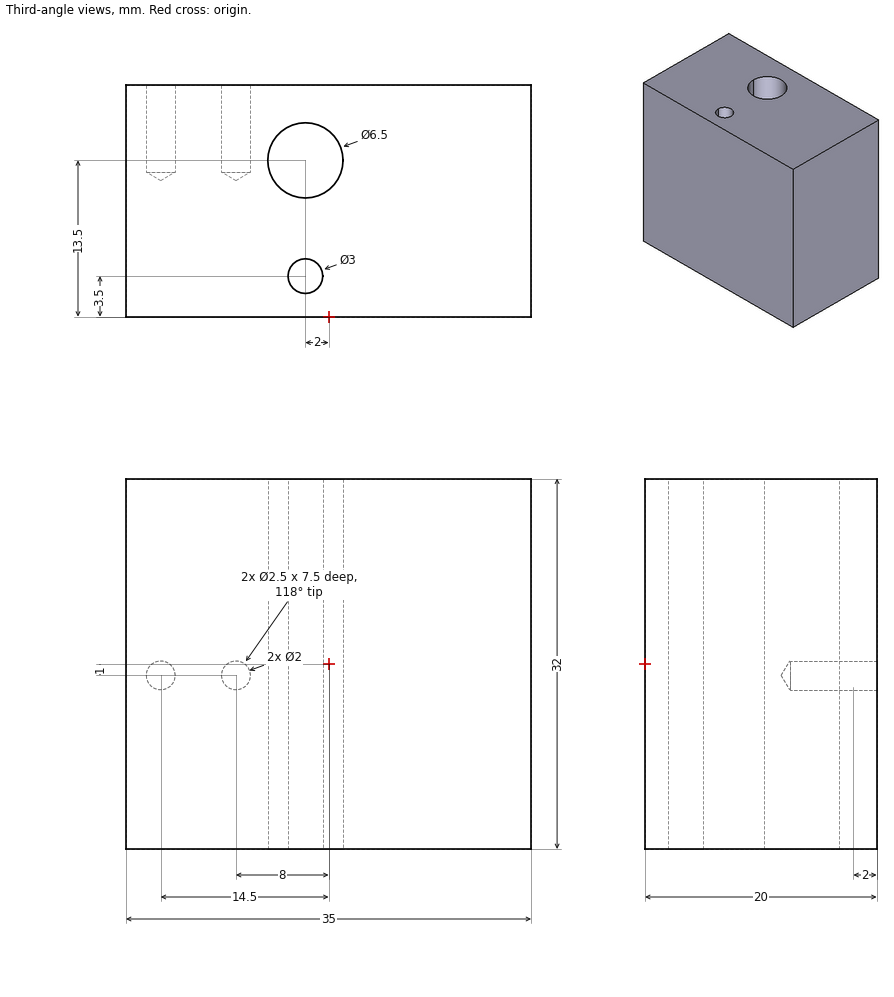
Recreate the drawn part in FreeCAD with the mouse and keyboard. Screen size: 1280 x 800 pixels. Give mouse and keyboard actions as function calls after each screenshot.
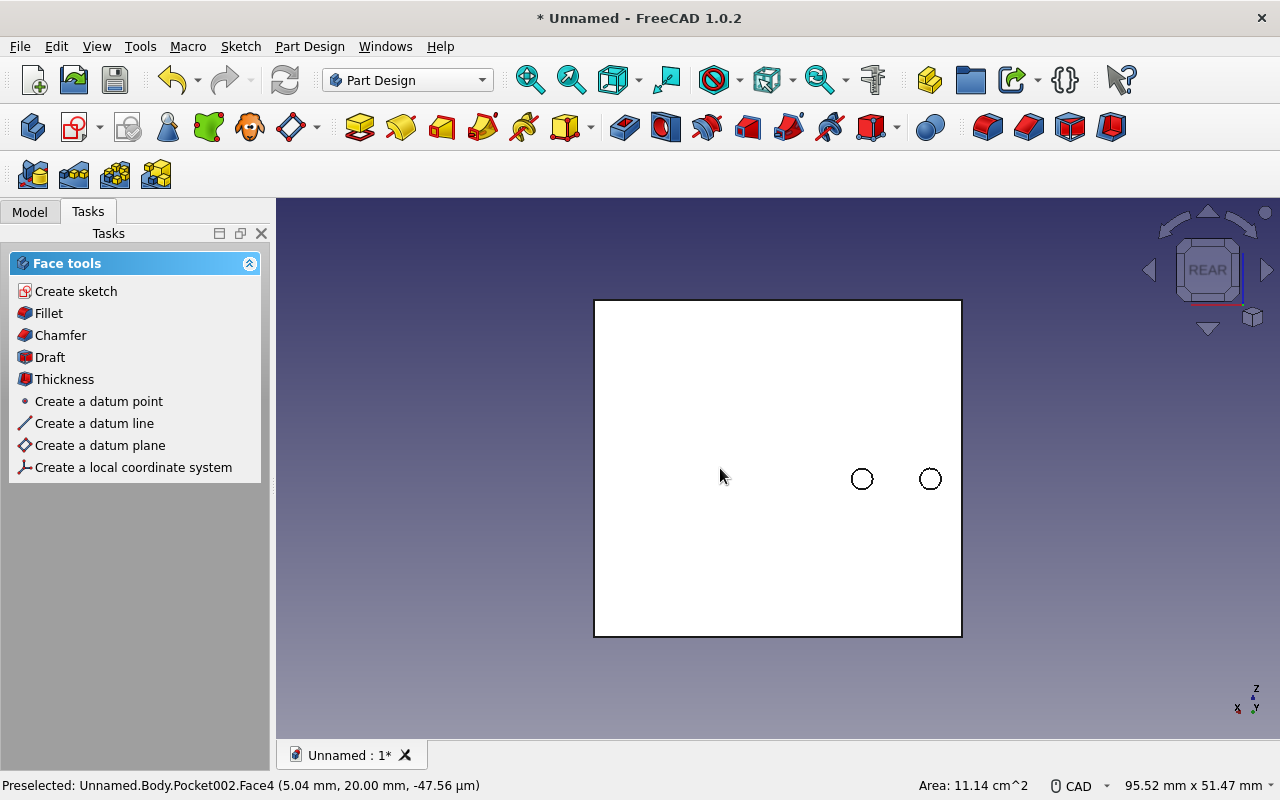
click(74, 128)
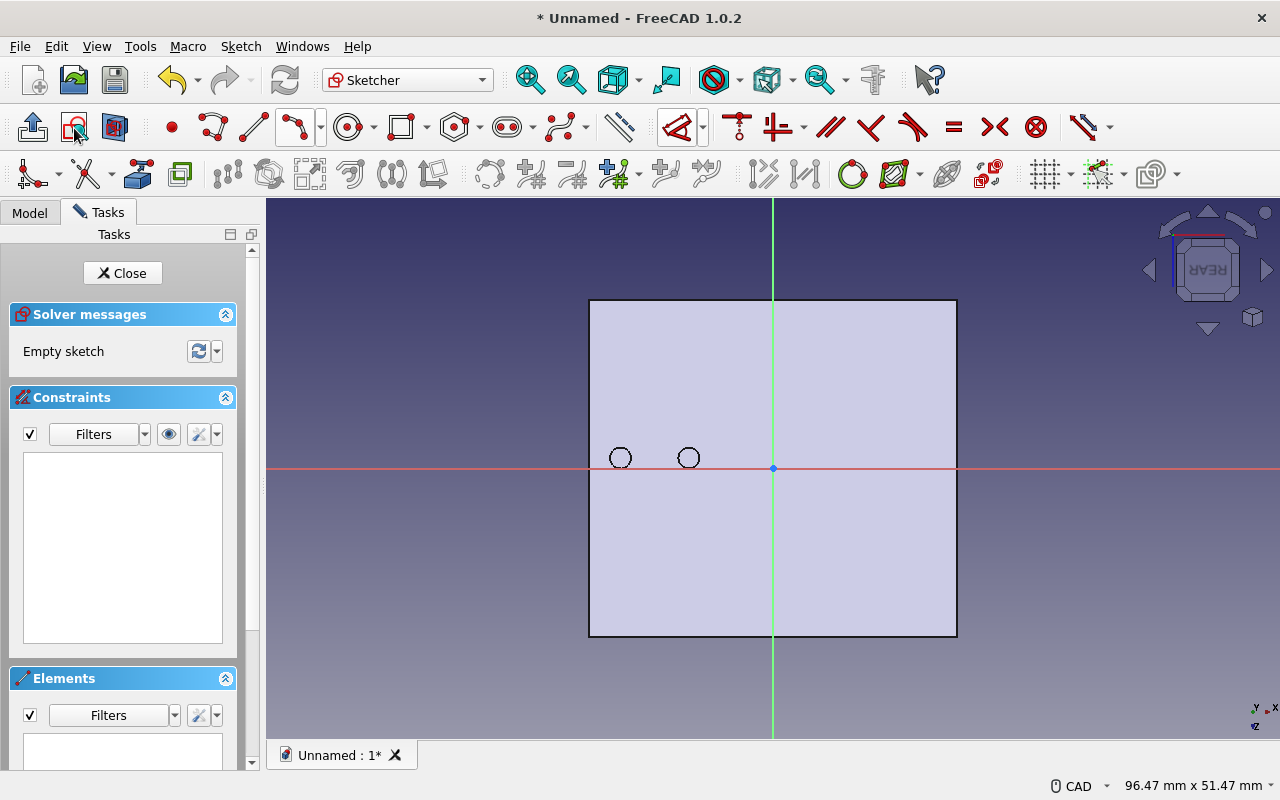
scroll(684, 453, up, 6)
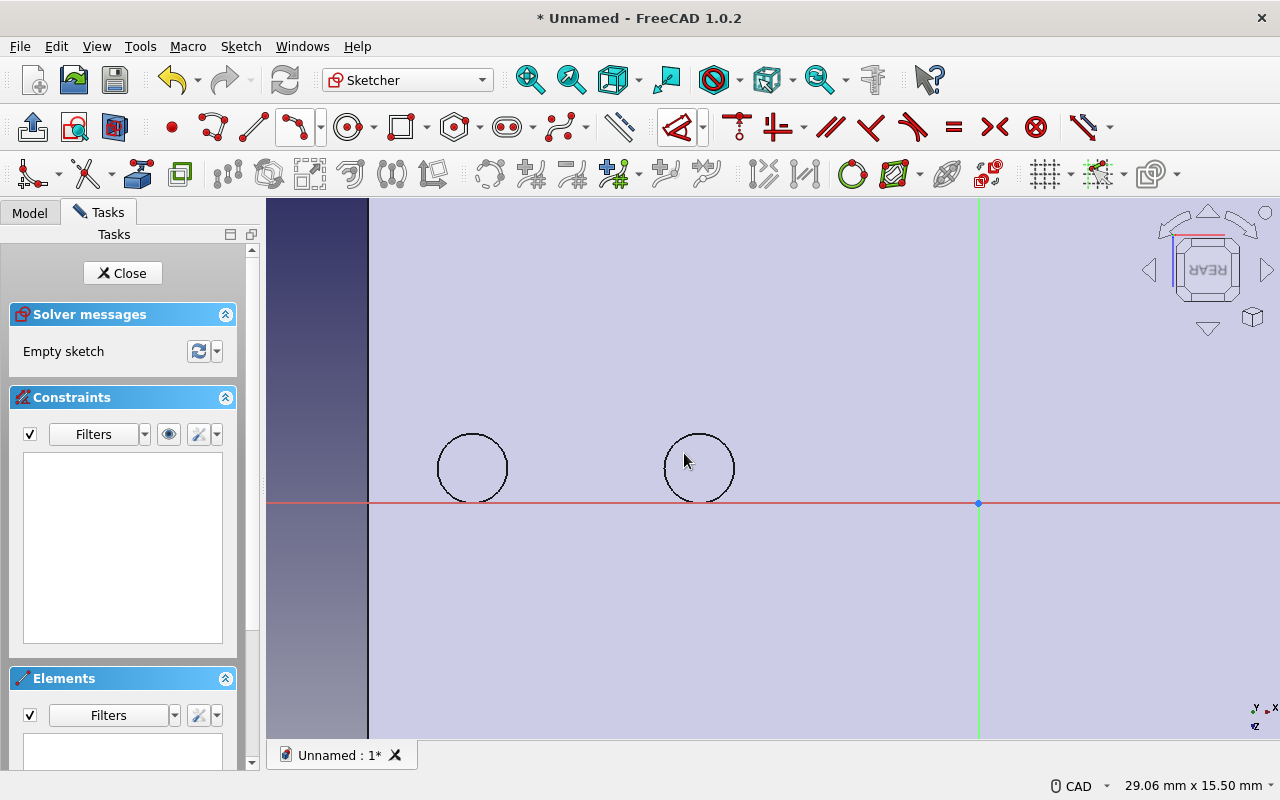
key(g)
key(c)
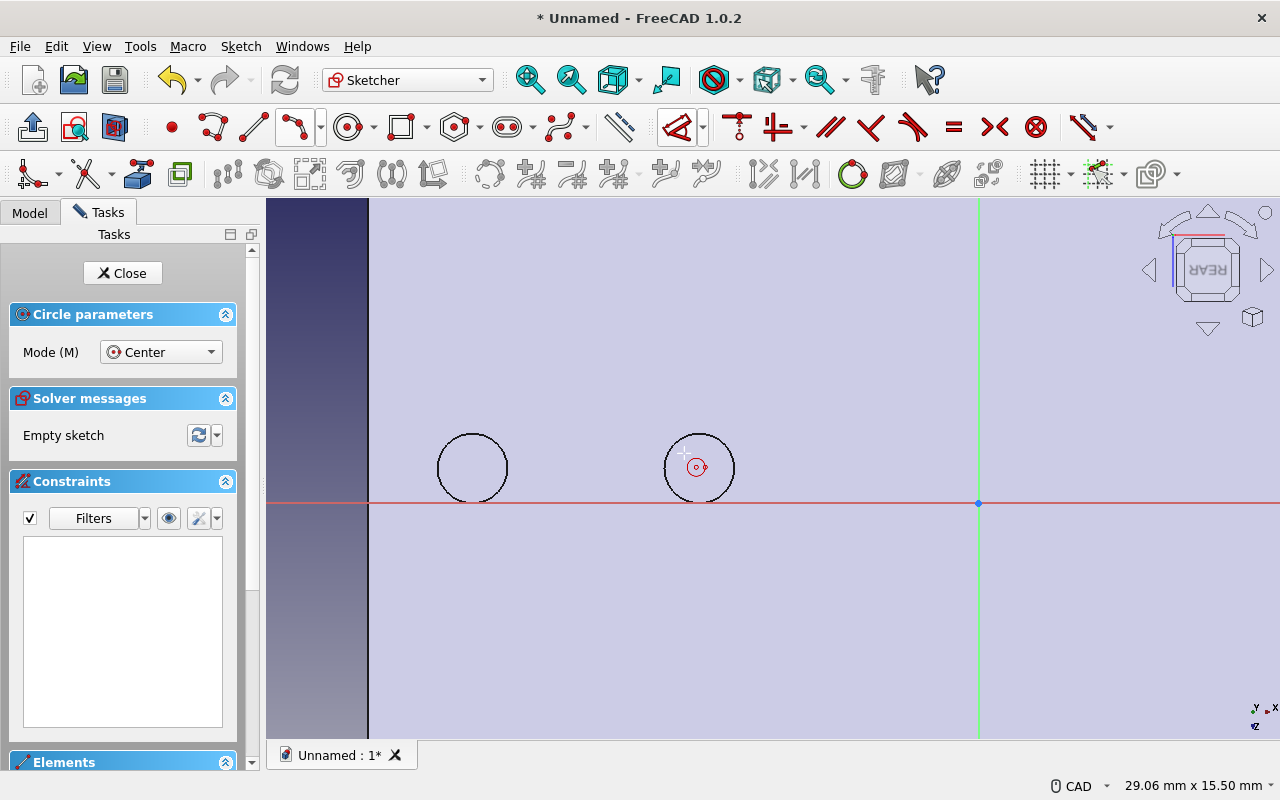
click(699, 468)
click(730, 438)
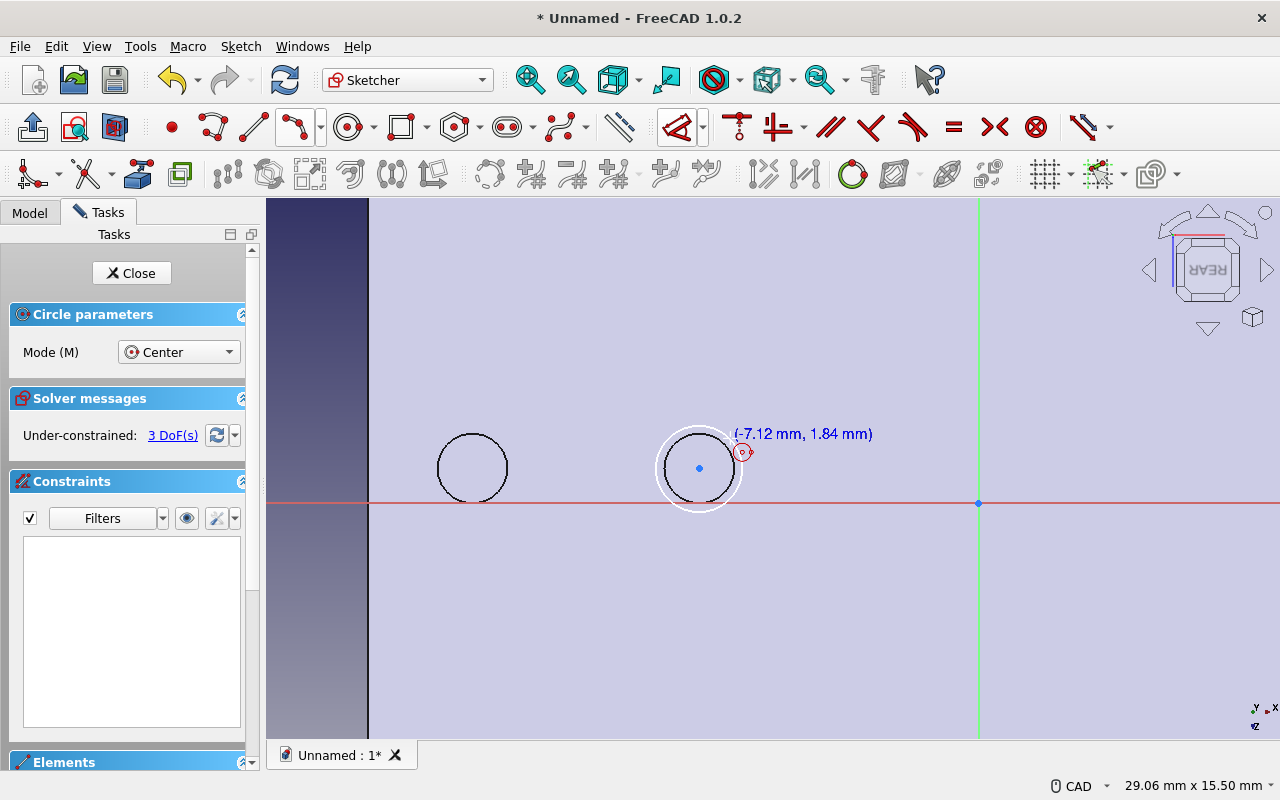
click(473, 468)
click(503, 438)
key(Escape)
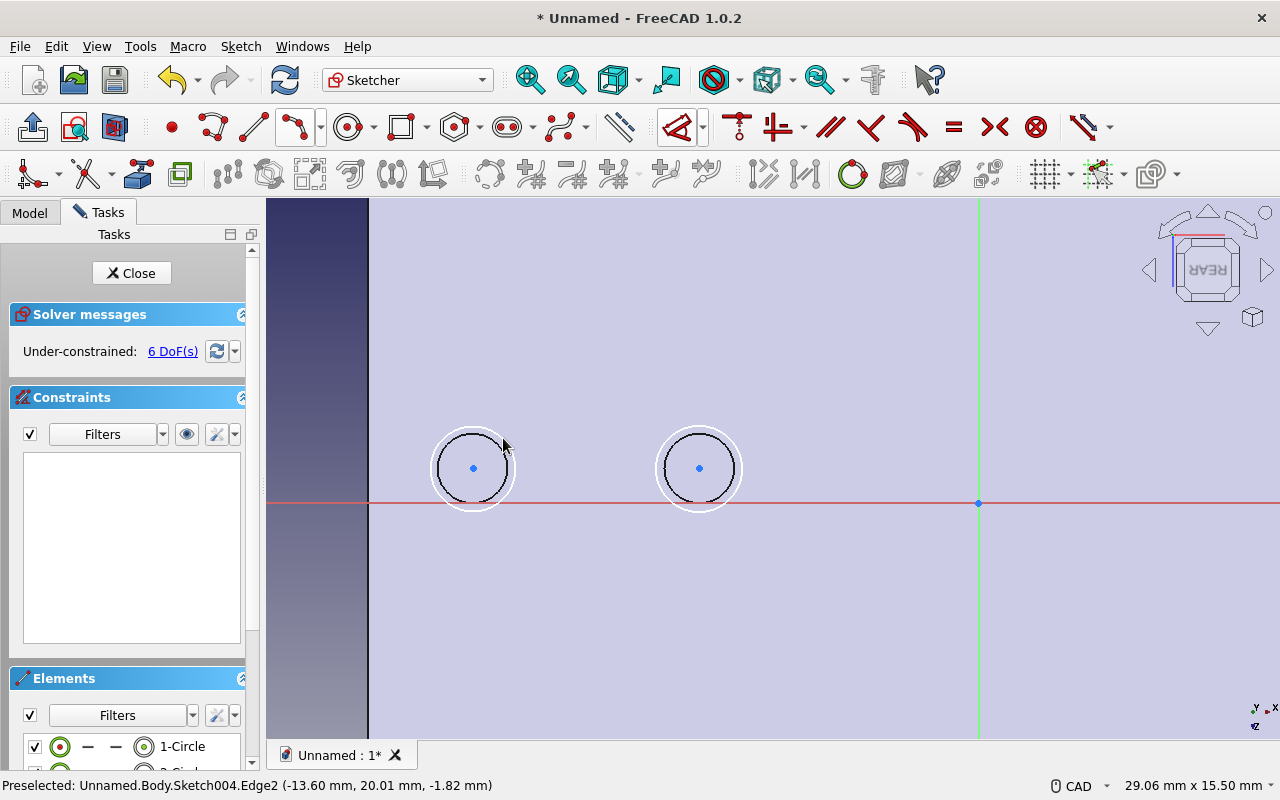
click(729, 438)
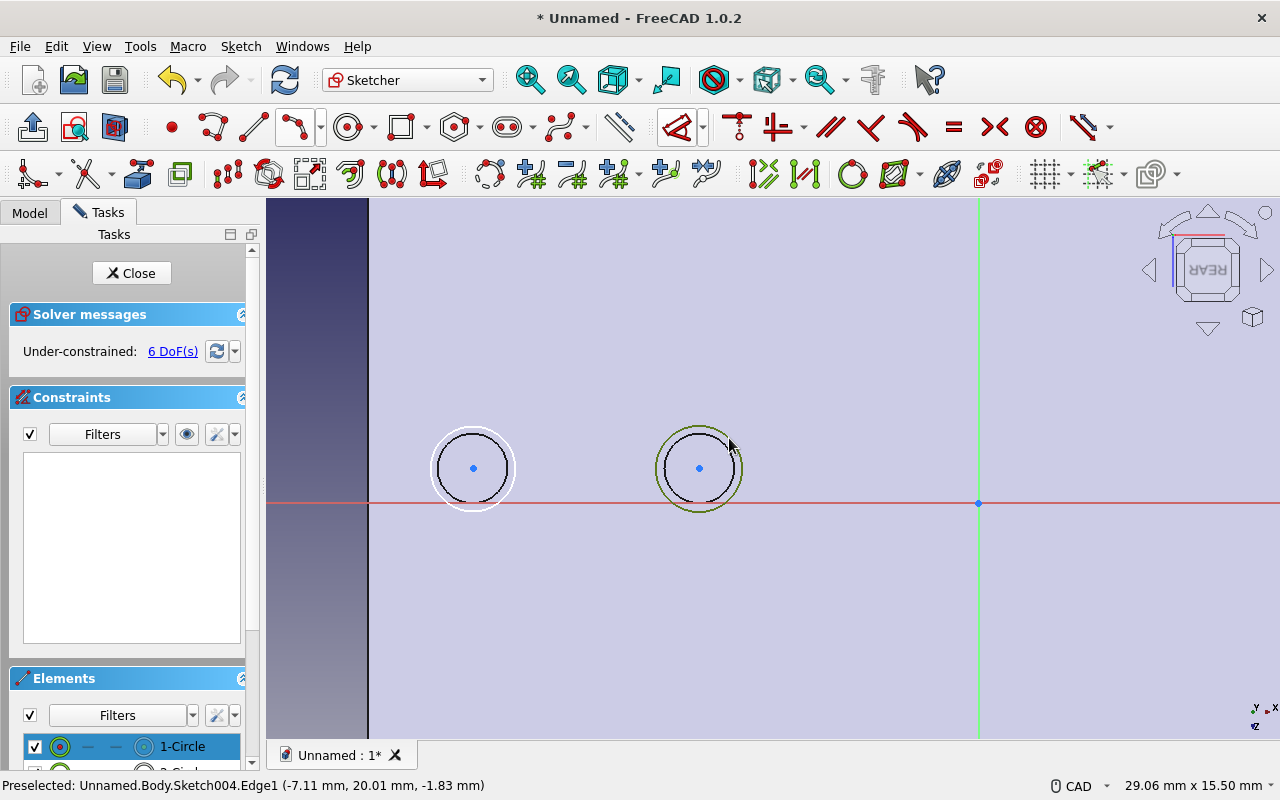
click(503, 439)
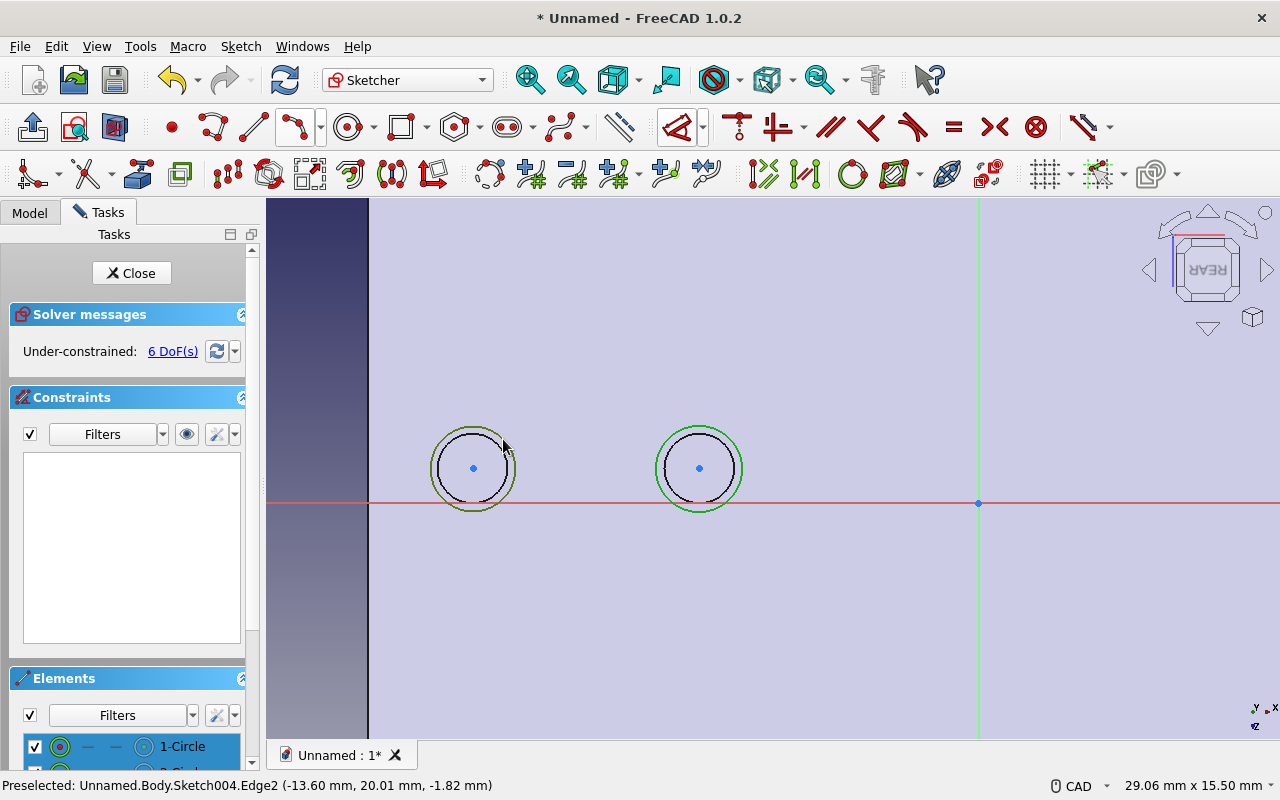
key(e)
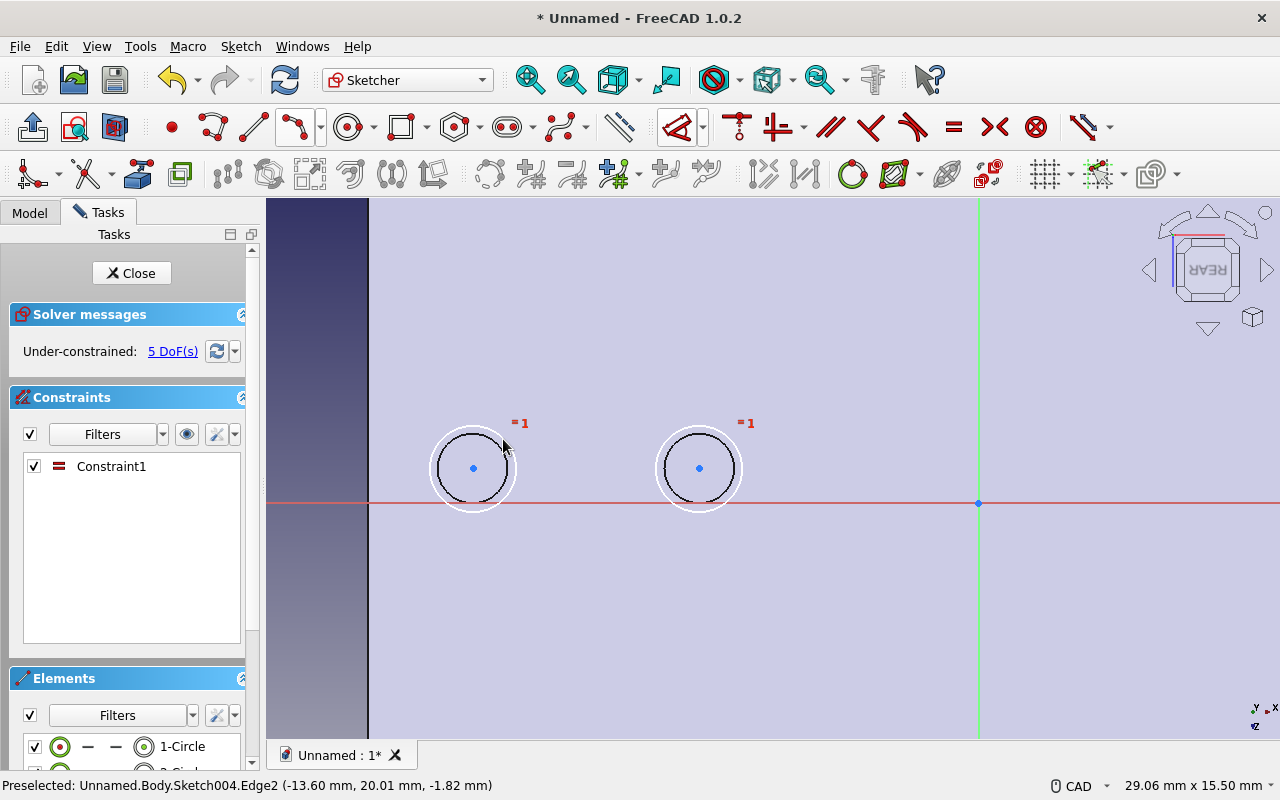
click(729, 438)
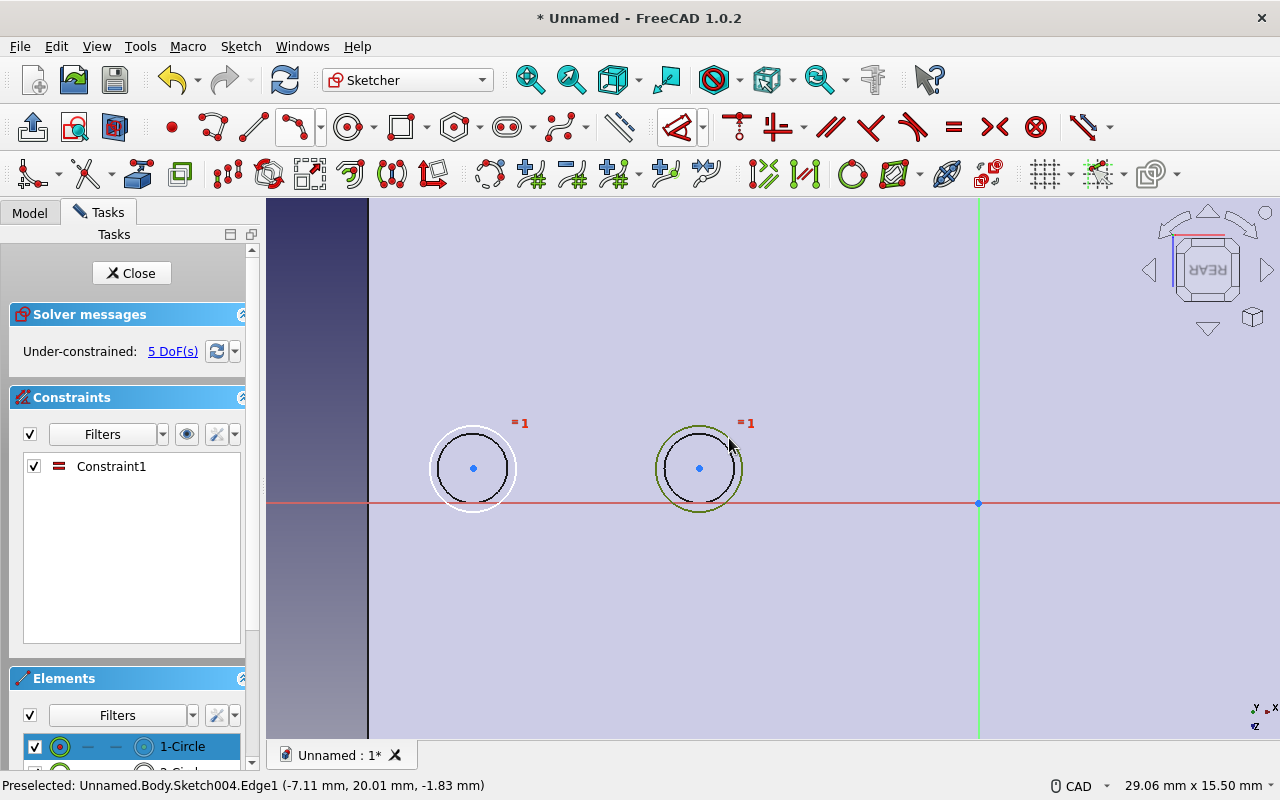
key(k)
key(o)